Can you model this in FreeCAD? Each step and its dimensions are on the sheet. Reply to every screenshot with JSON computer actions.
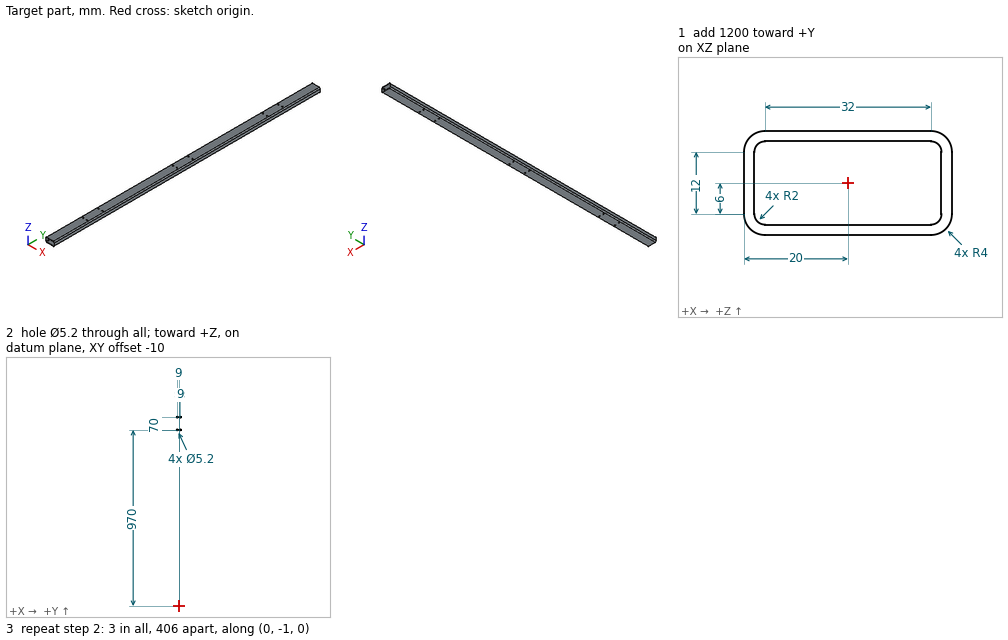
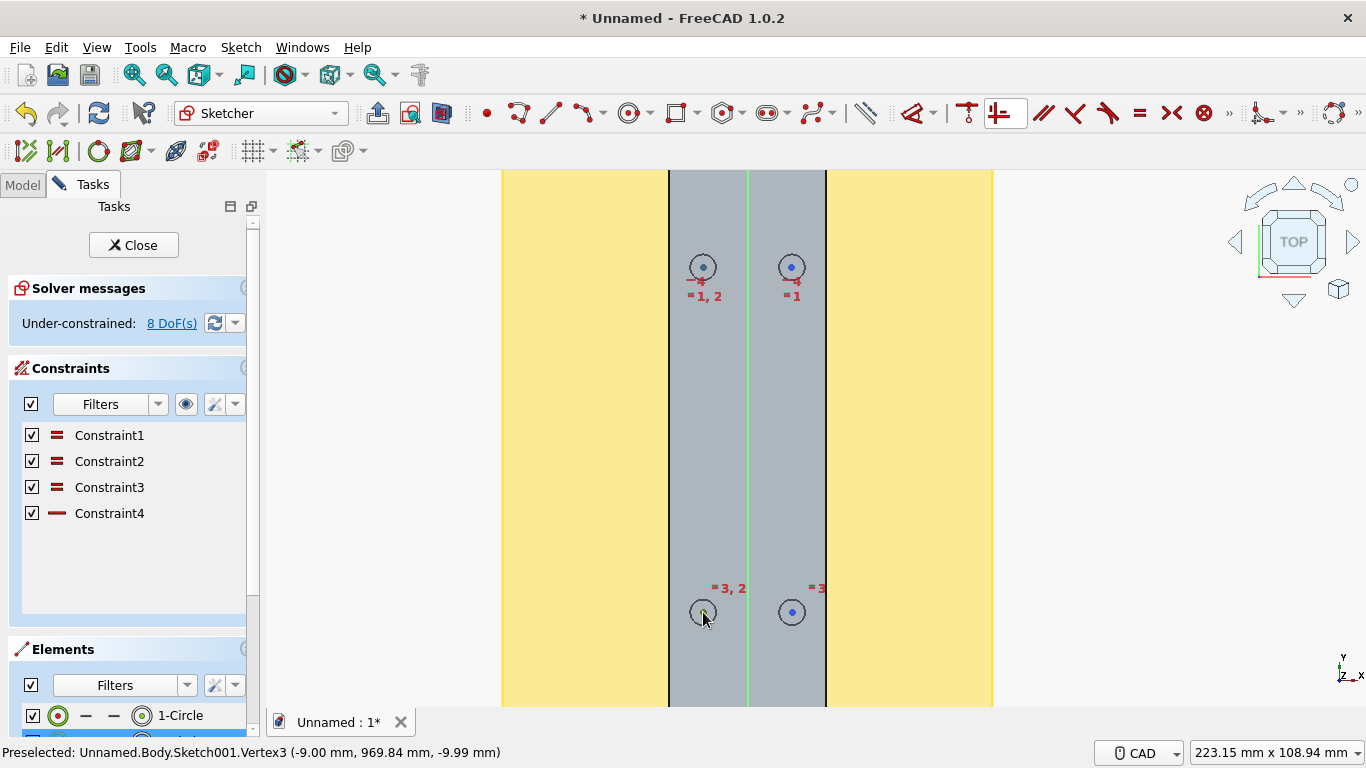
{"action": "key", "text": "v"}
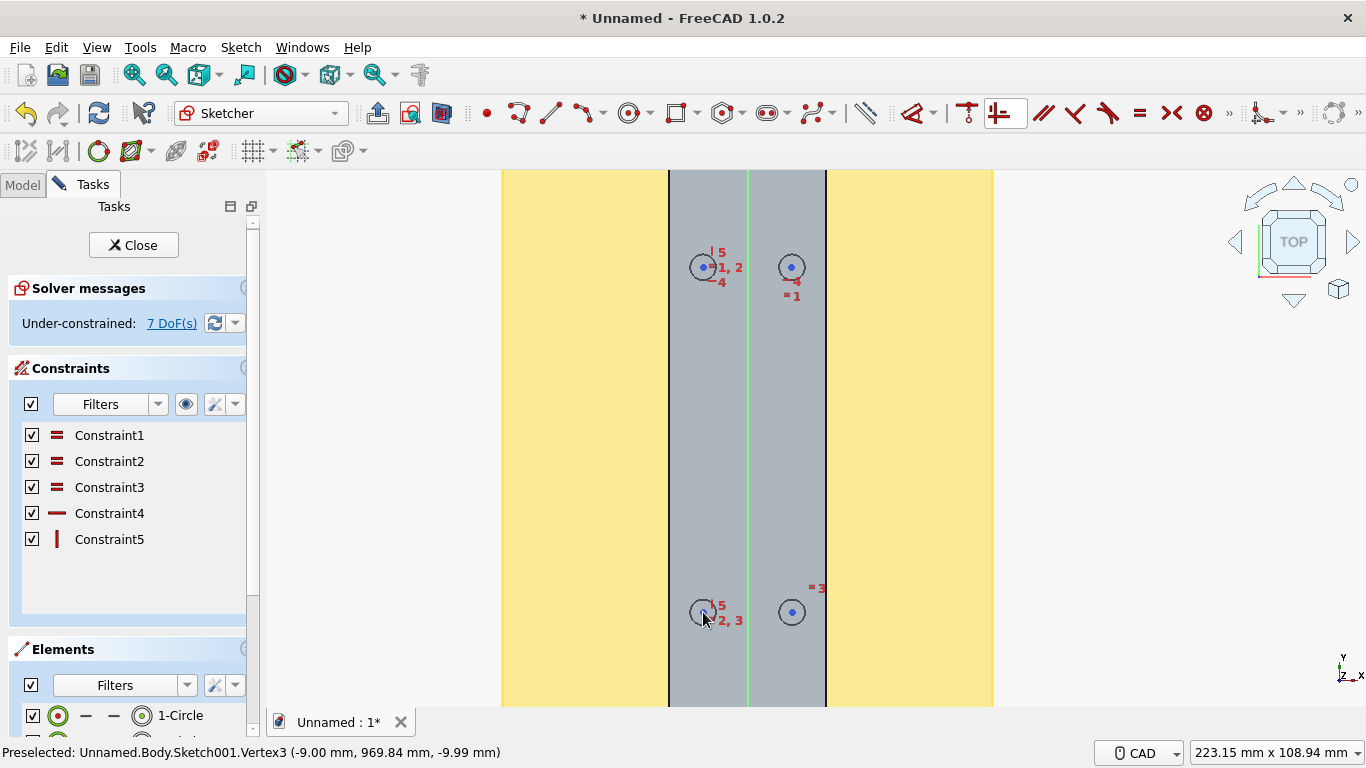
{"action": "left_click", "coordinate": [792, 267]}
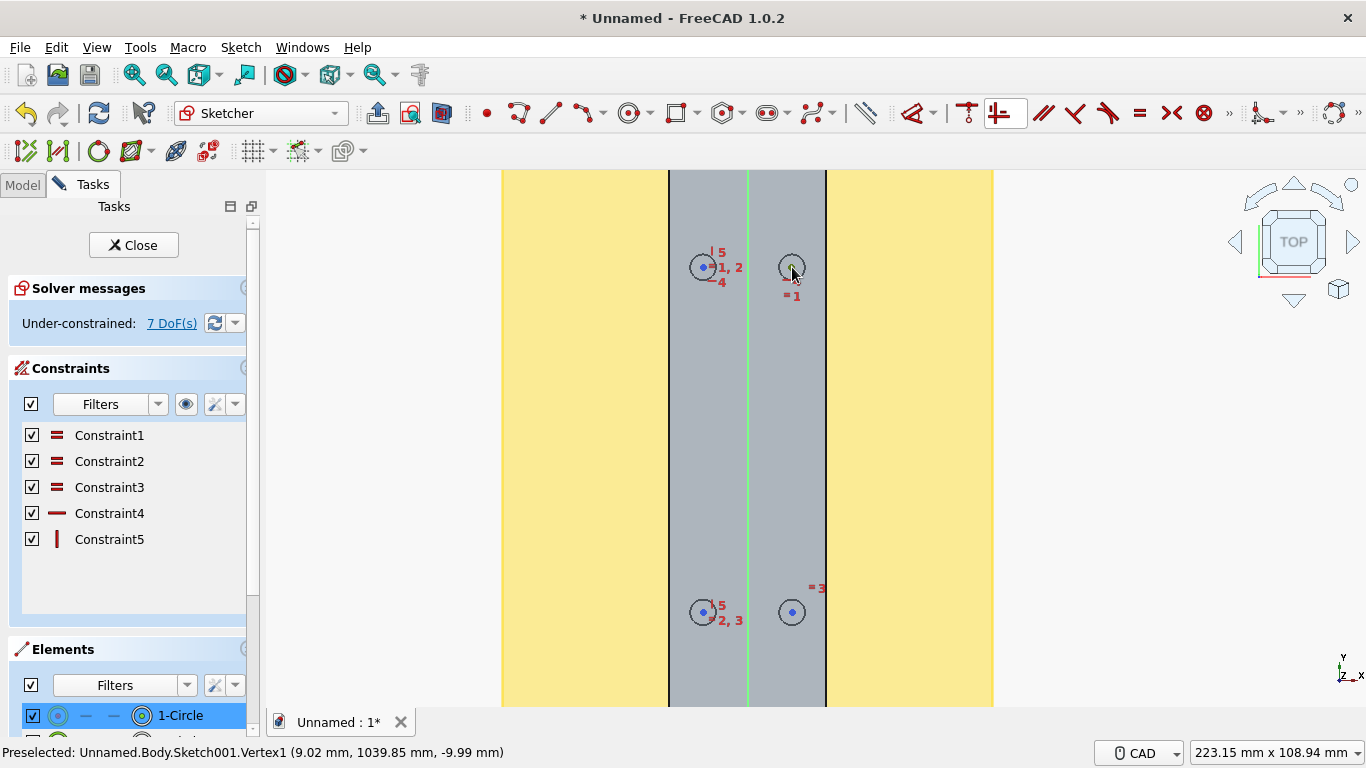
{"action": "left_click", "coordinate": [792, 612]}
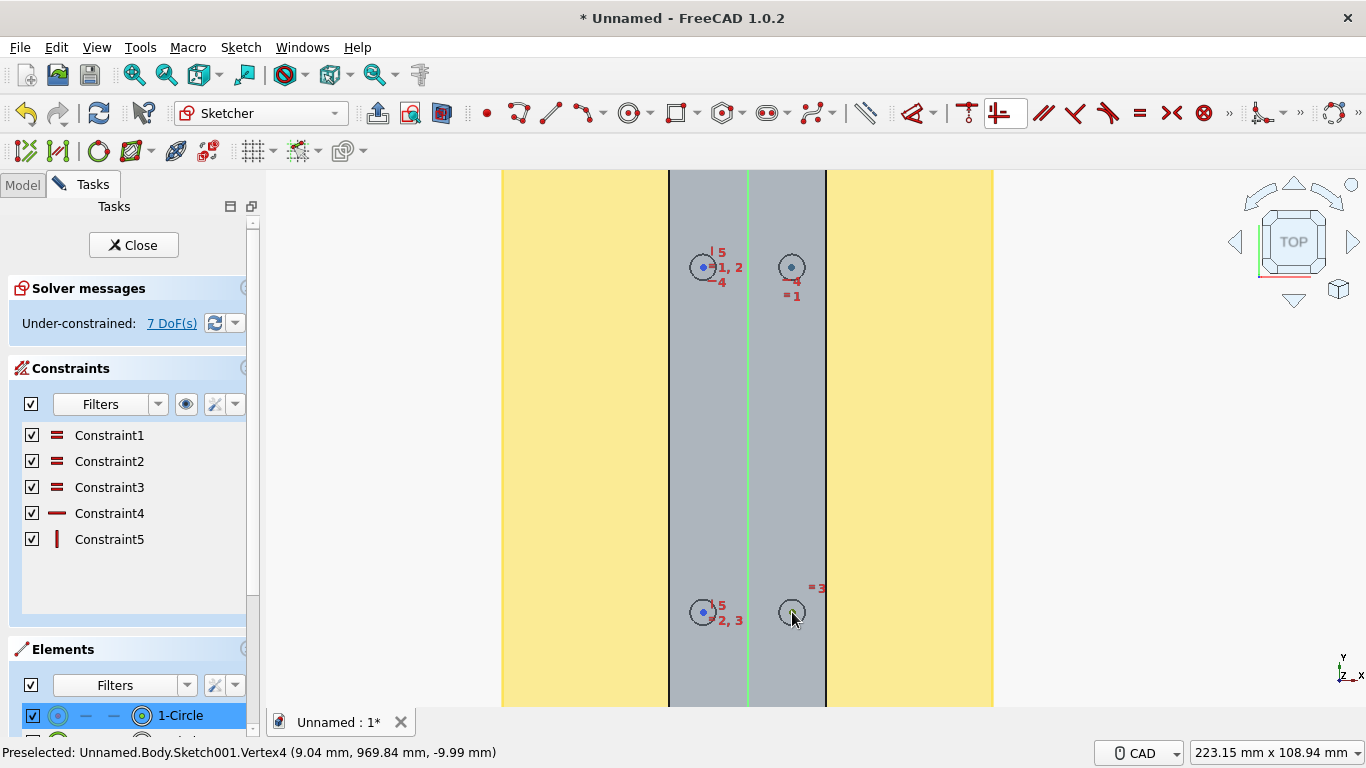
{"action": "key", "text": "v"}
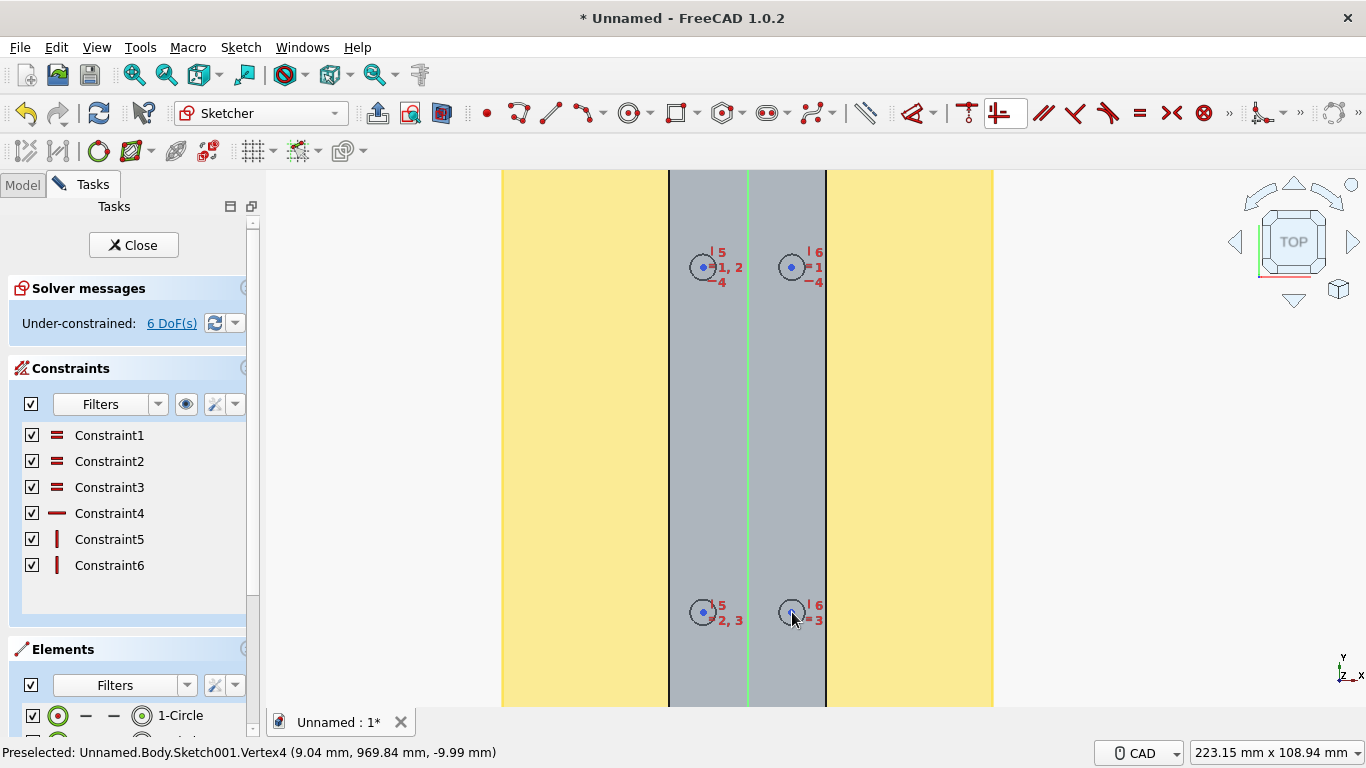
{"action": "left_click", "coordinate": [703, 612]}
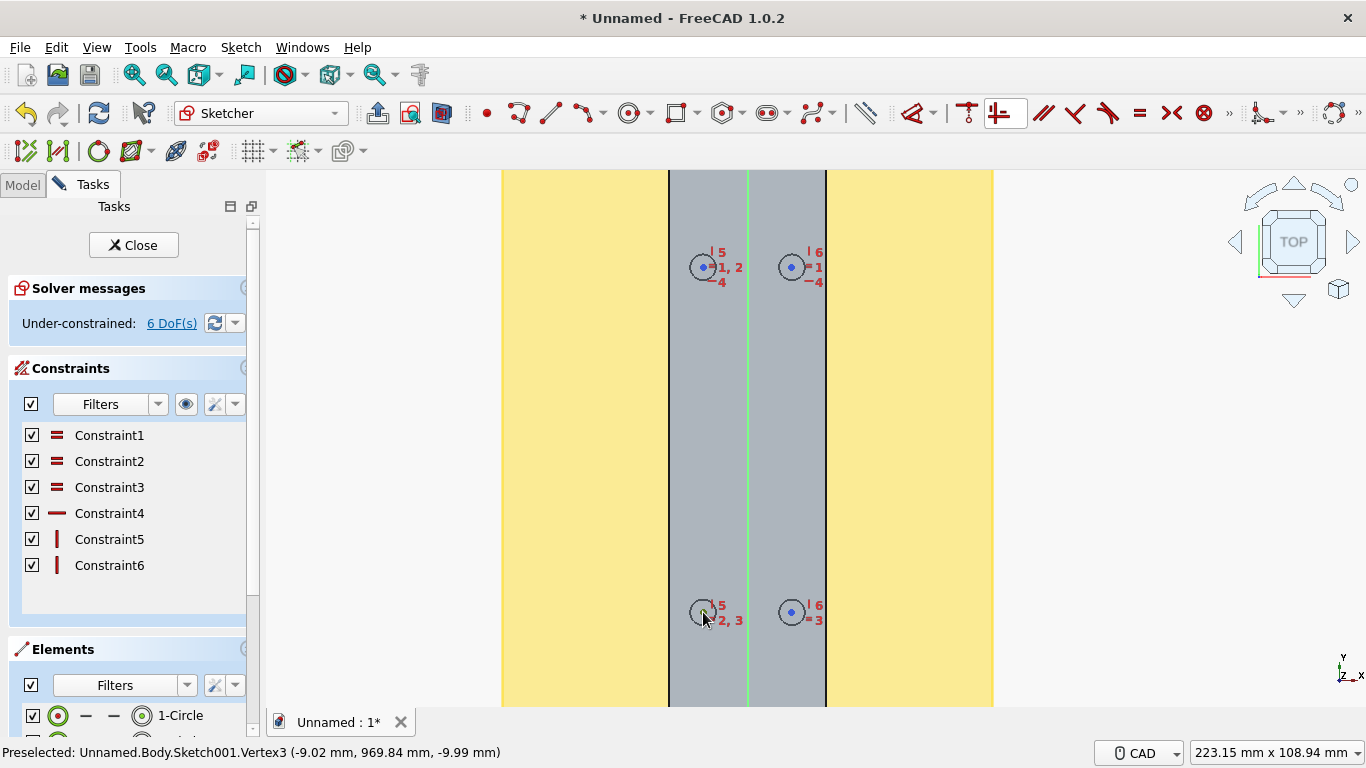
{"action": "left_click", "coordinate": [792, 612]}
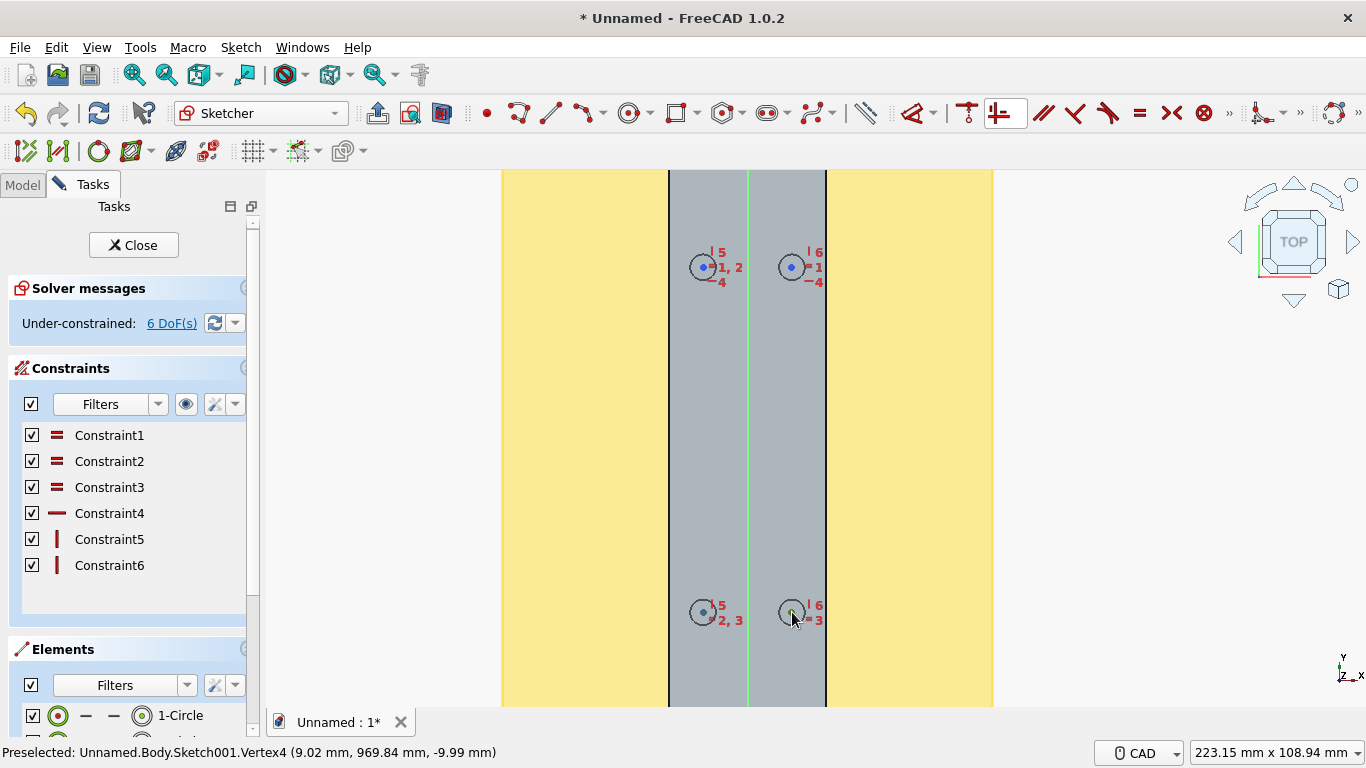
{"action": "key", "text": "h"}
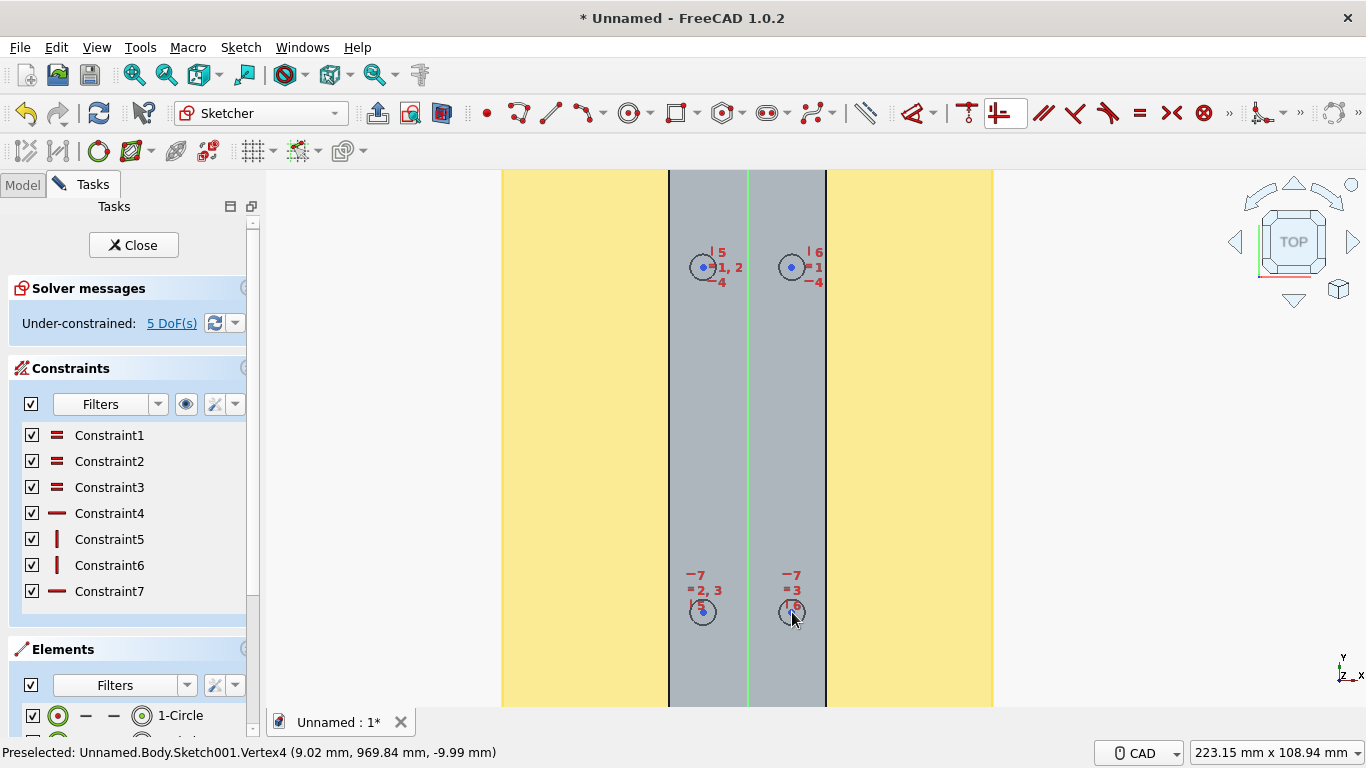
{"action": "key", "text": "d"}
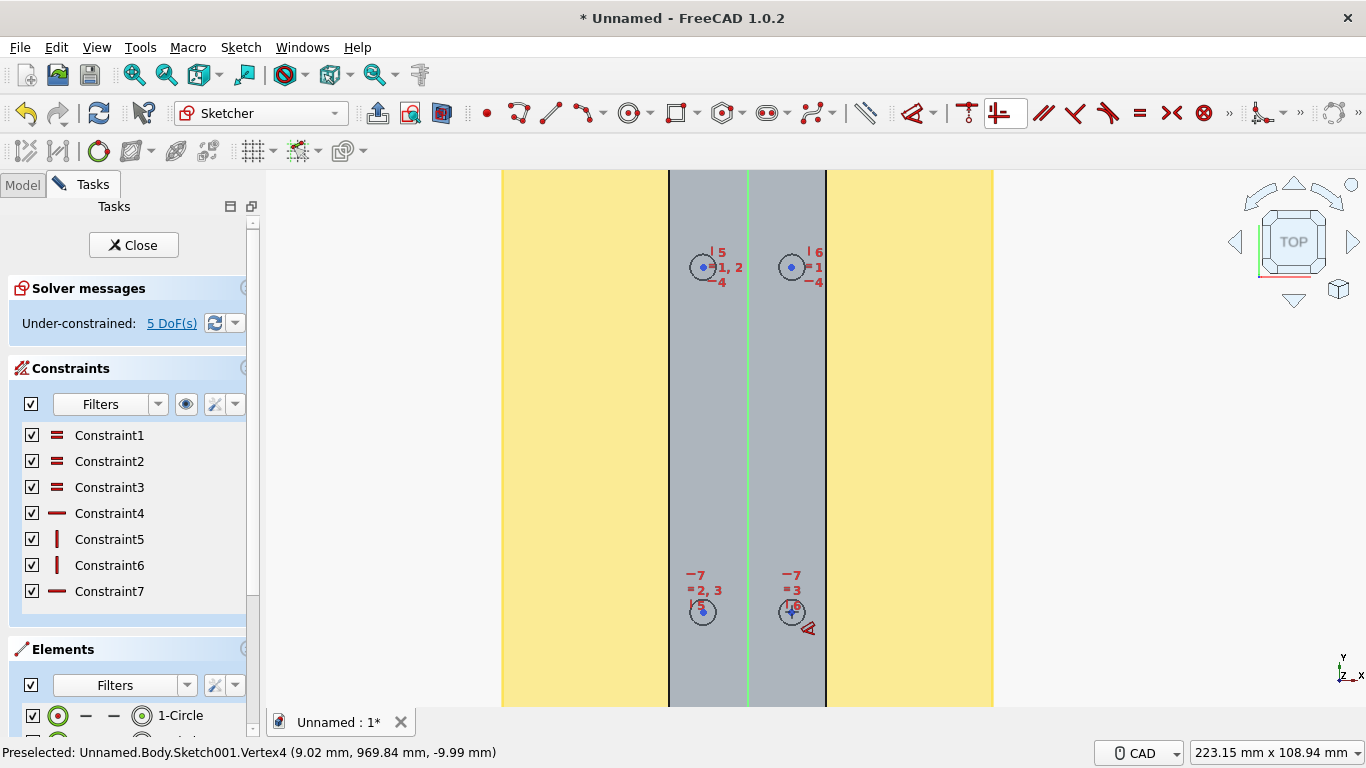
{"action": "scroll", "coordinate": [801, 258], "scroll_direction": "up", "scroll_amount": 3}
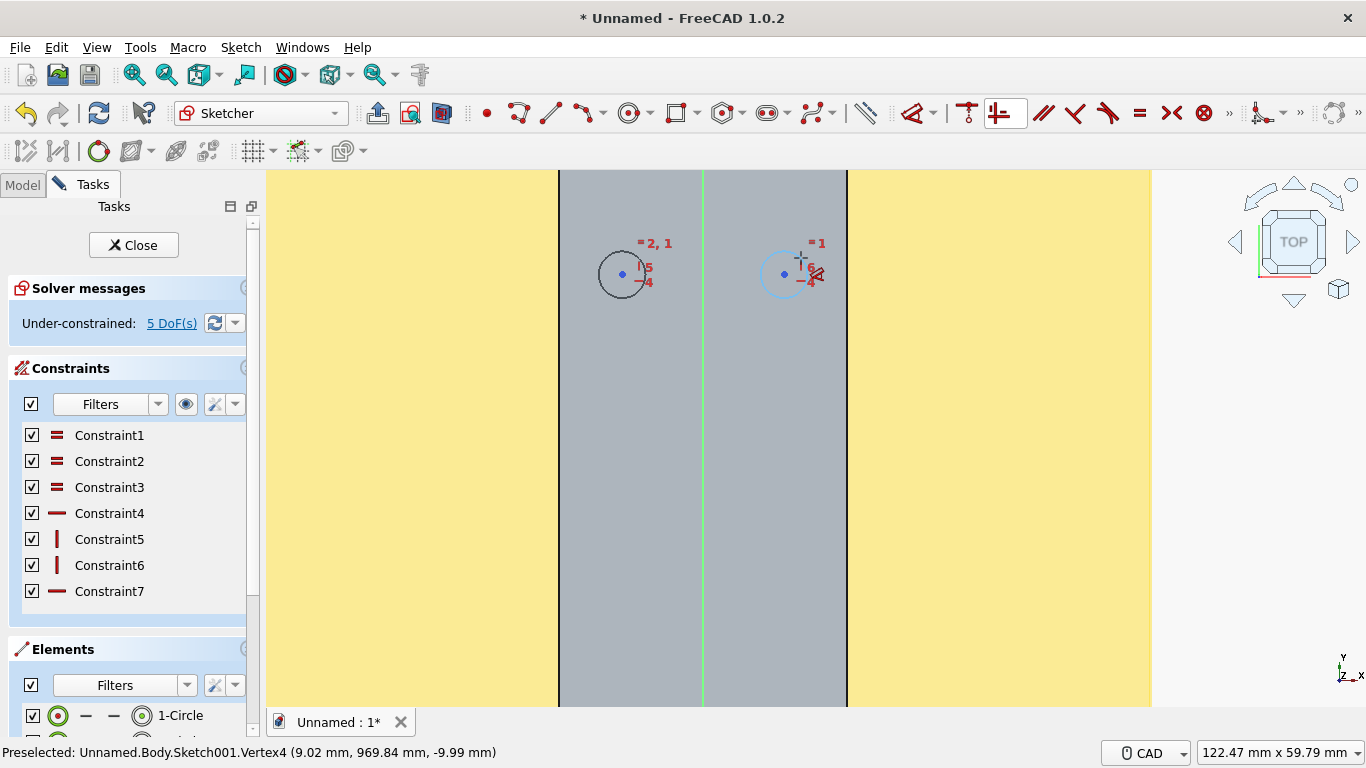
{"action": "left_click", "coordinate": [801, 258]}
{"action": "left_click", "coordinate": [824, 235]}